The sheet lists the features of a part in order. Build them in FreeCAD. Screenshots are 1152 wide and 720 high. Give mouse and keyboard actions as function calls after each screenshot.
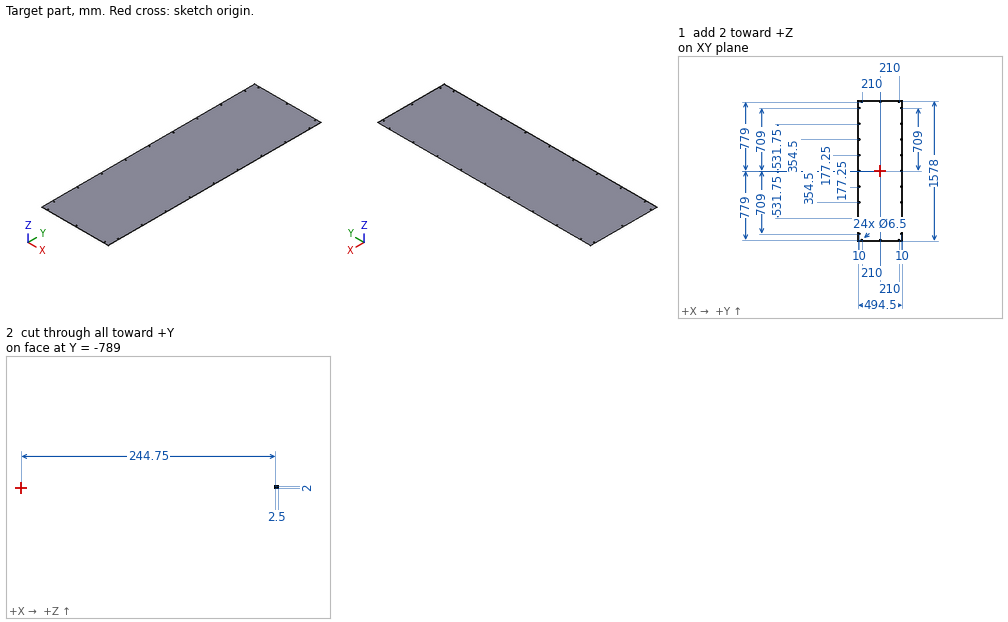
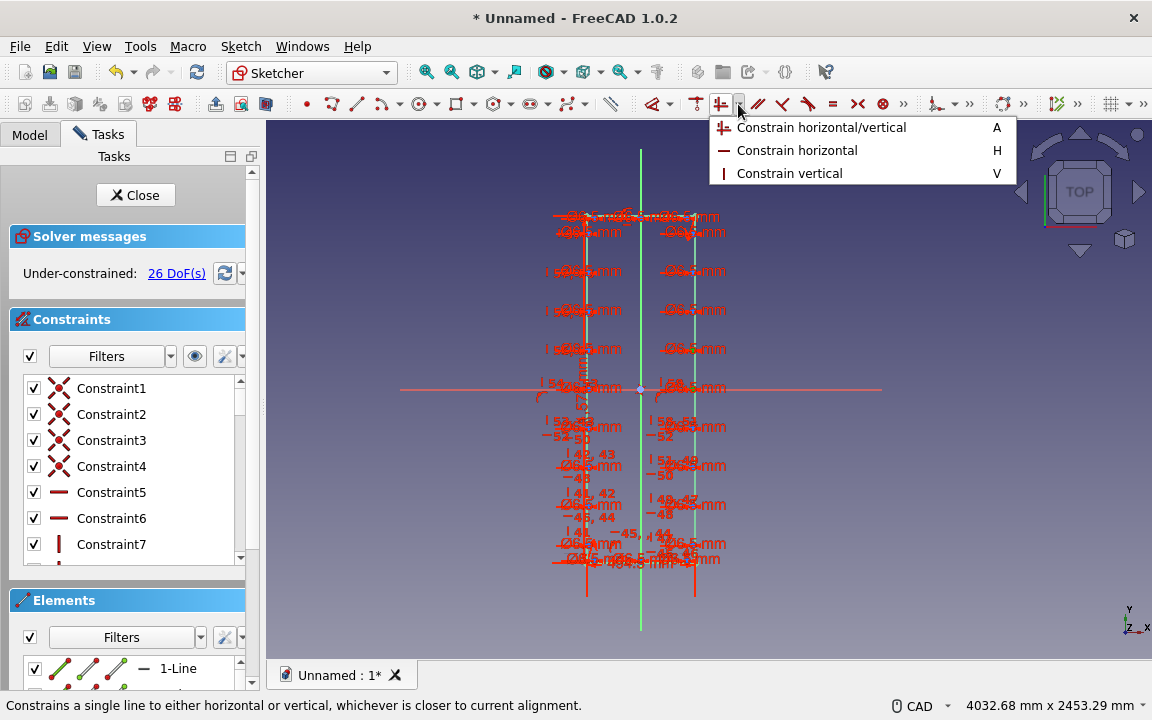
click(863, 174)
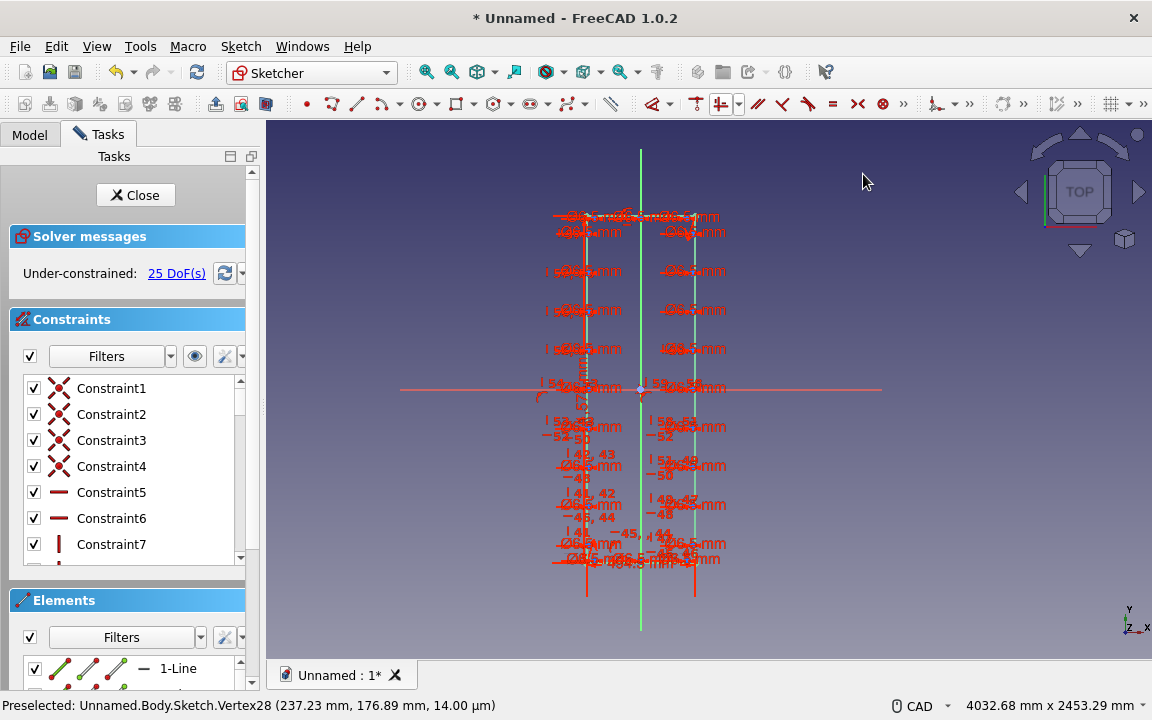
click(589, 351)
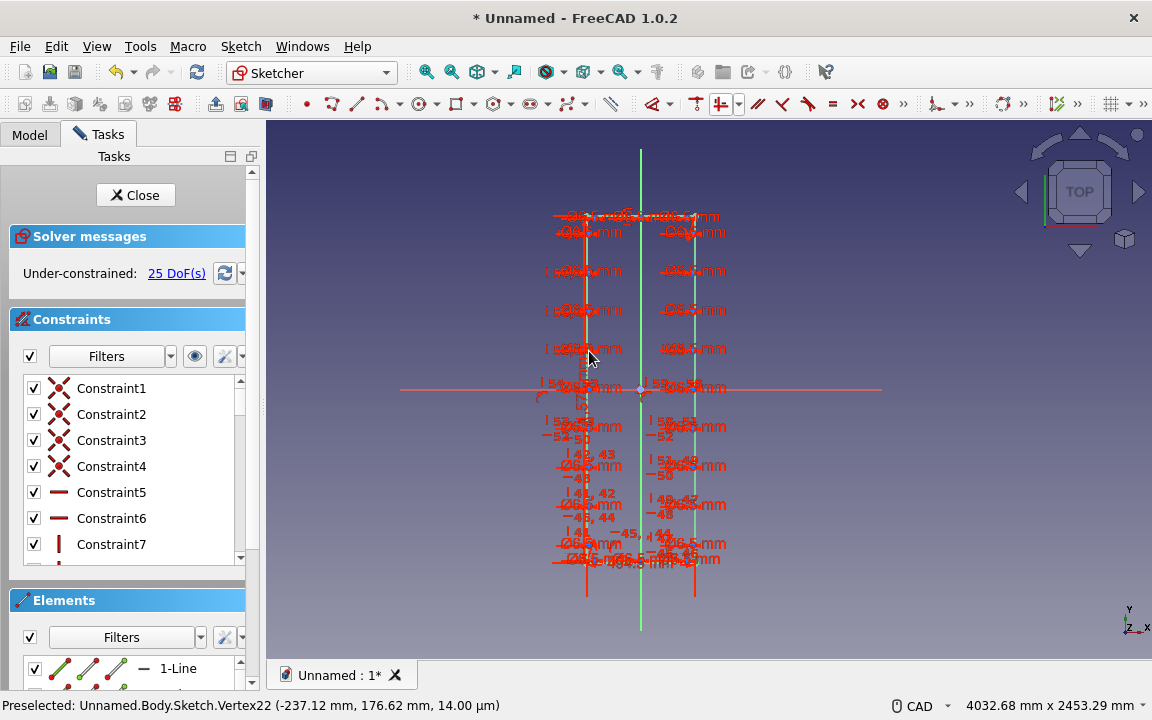
click(693, 351)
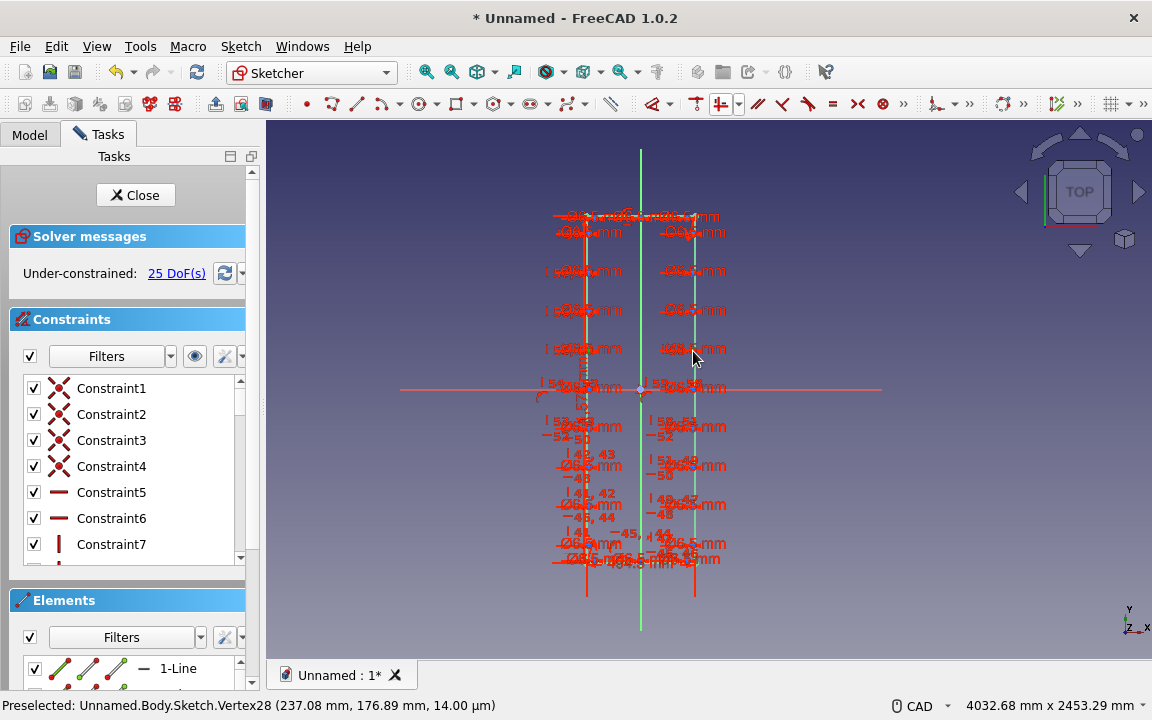
key(h)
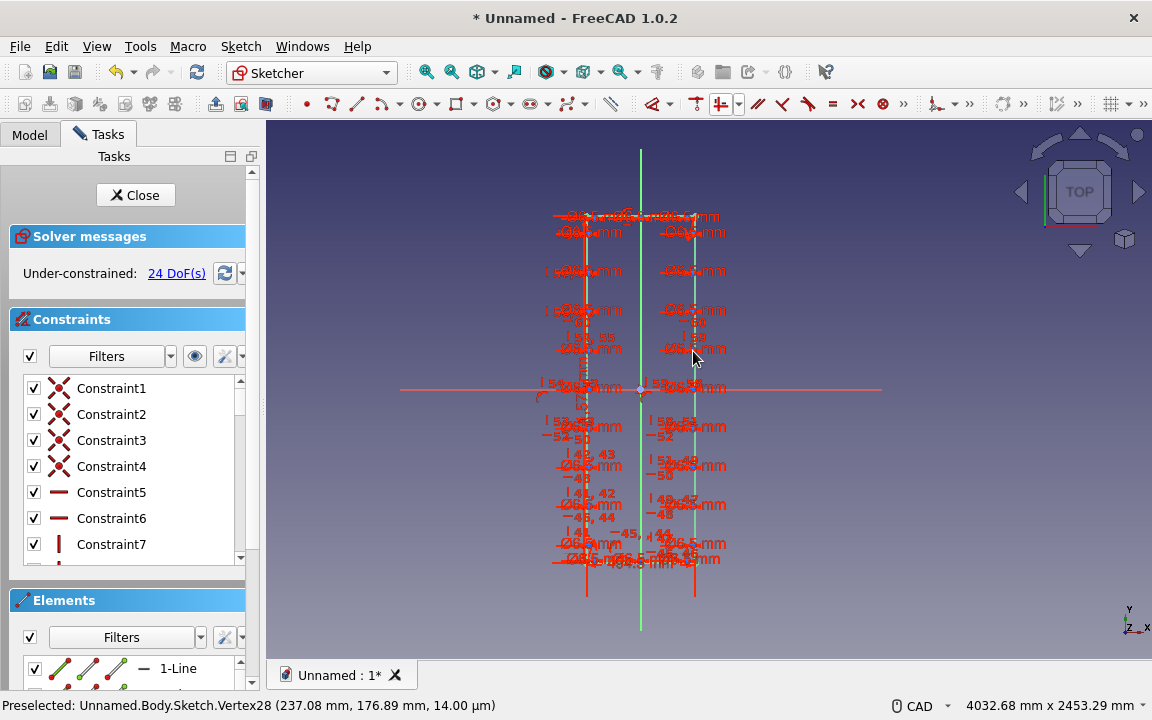
click(693, 351)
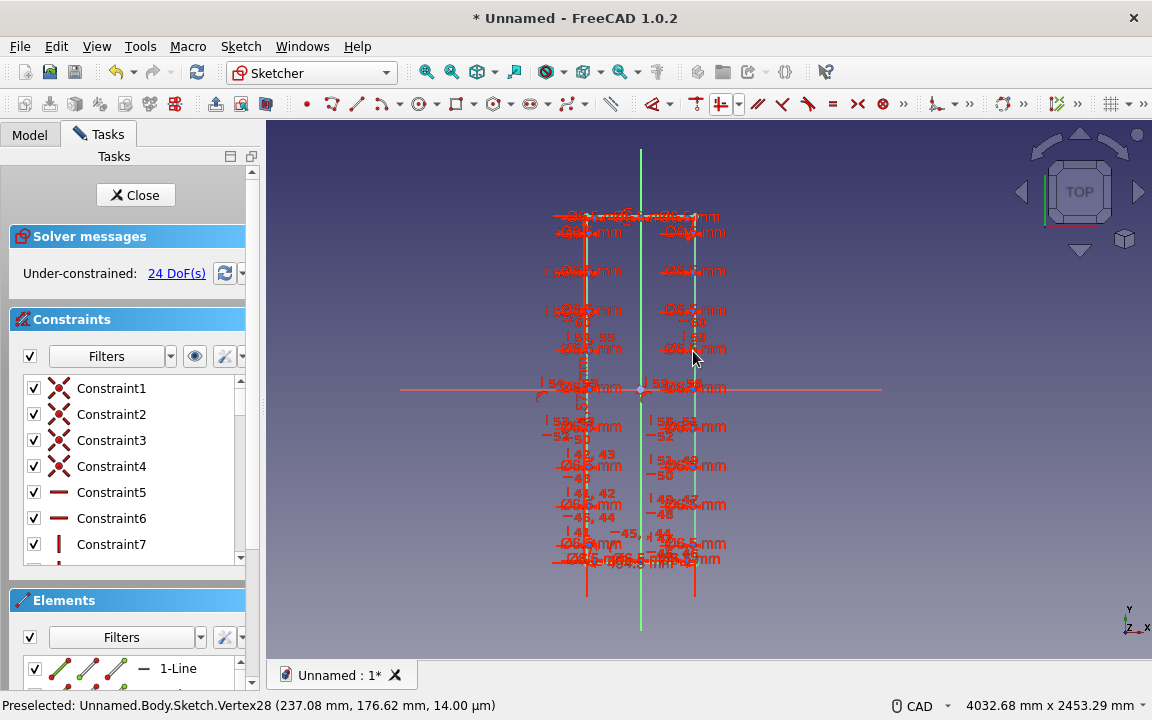
click(693, 312)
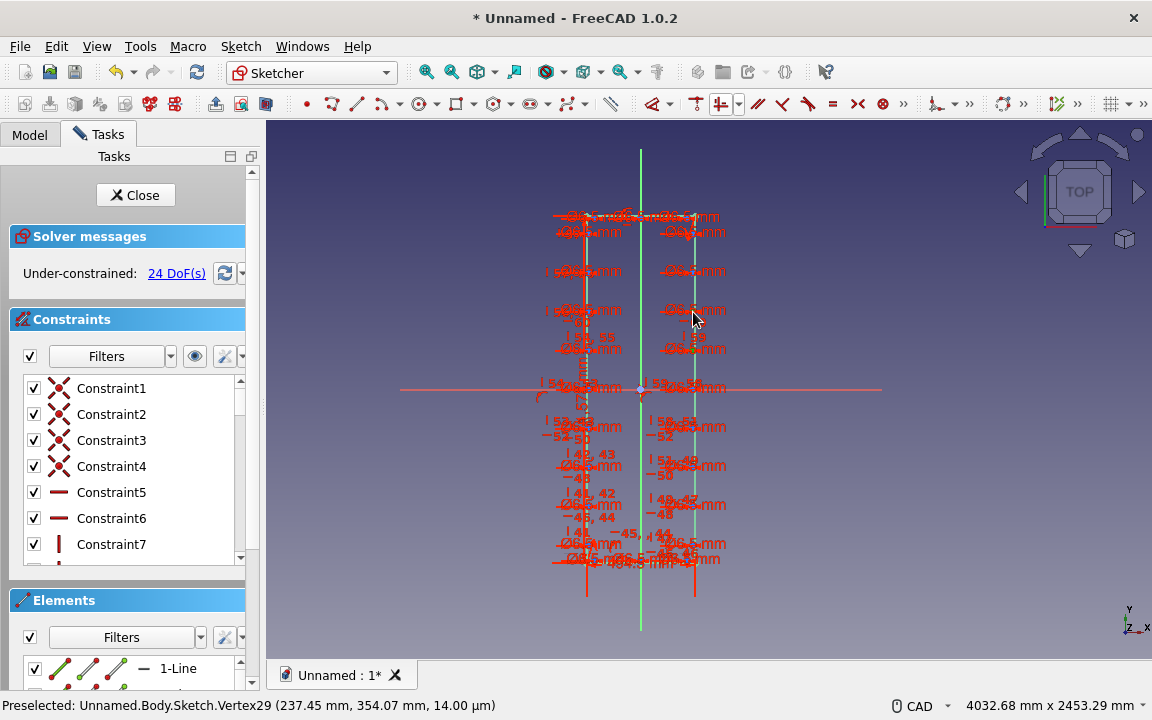
click(738, 104)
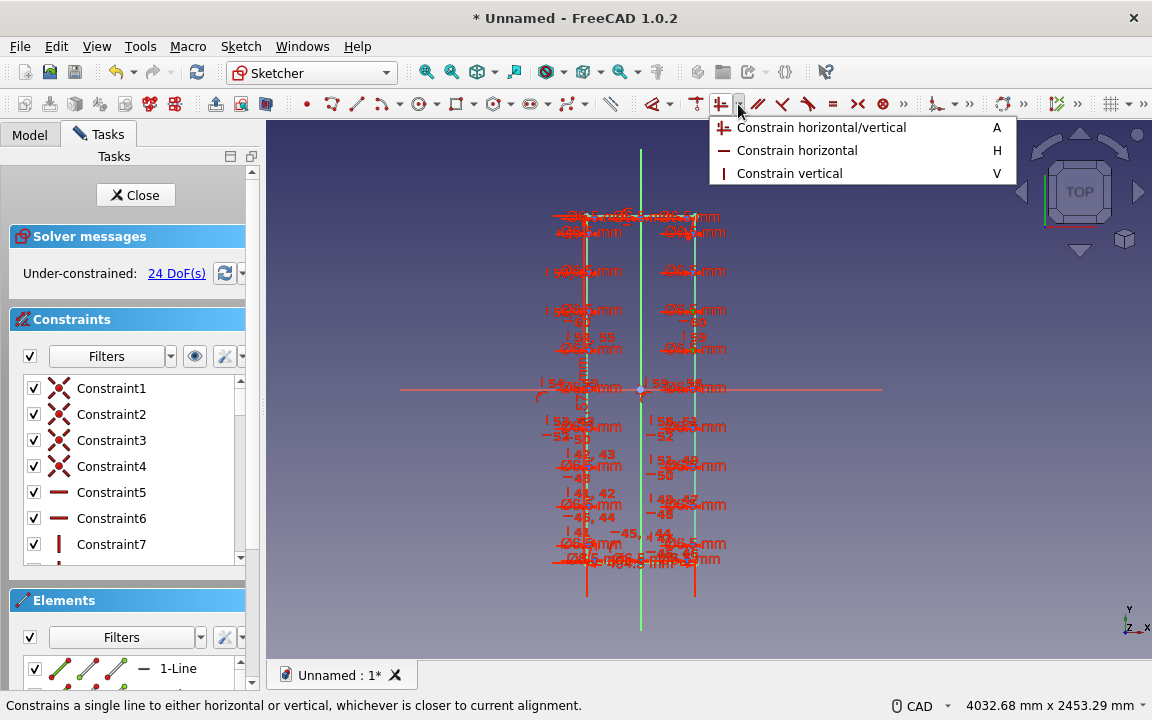
click(863, 174)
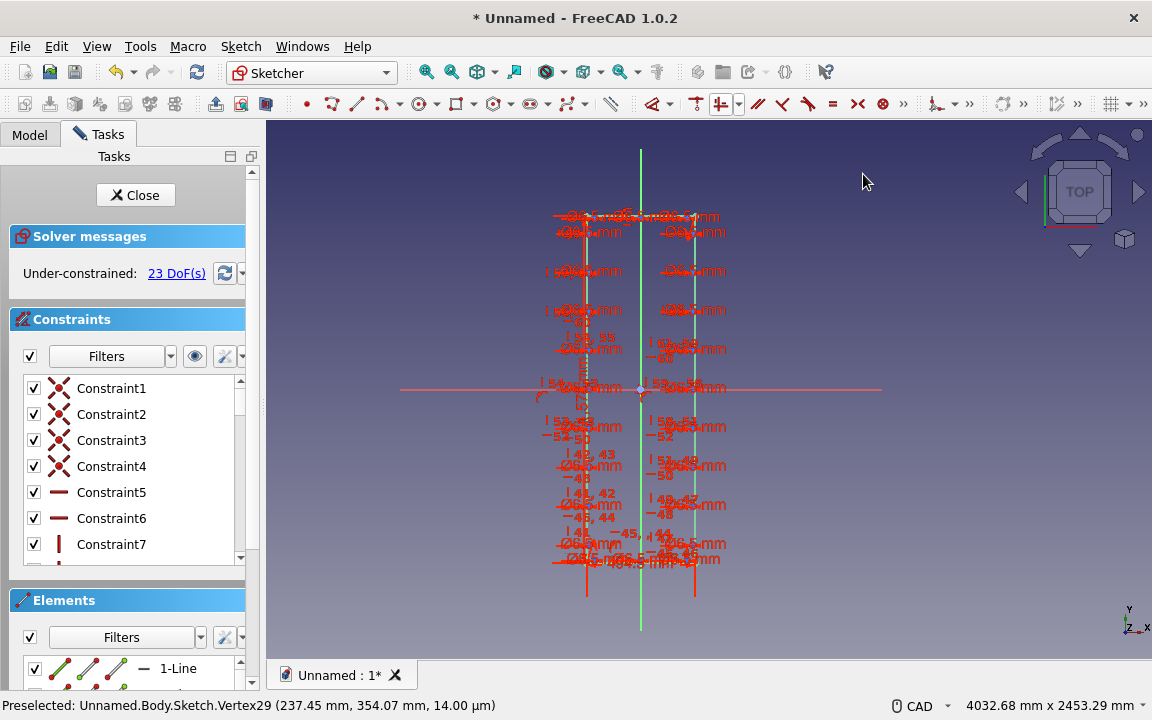
click(589, 312)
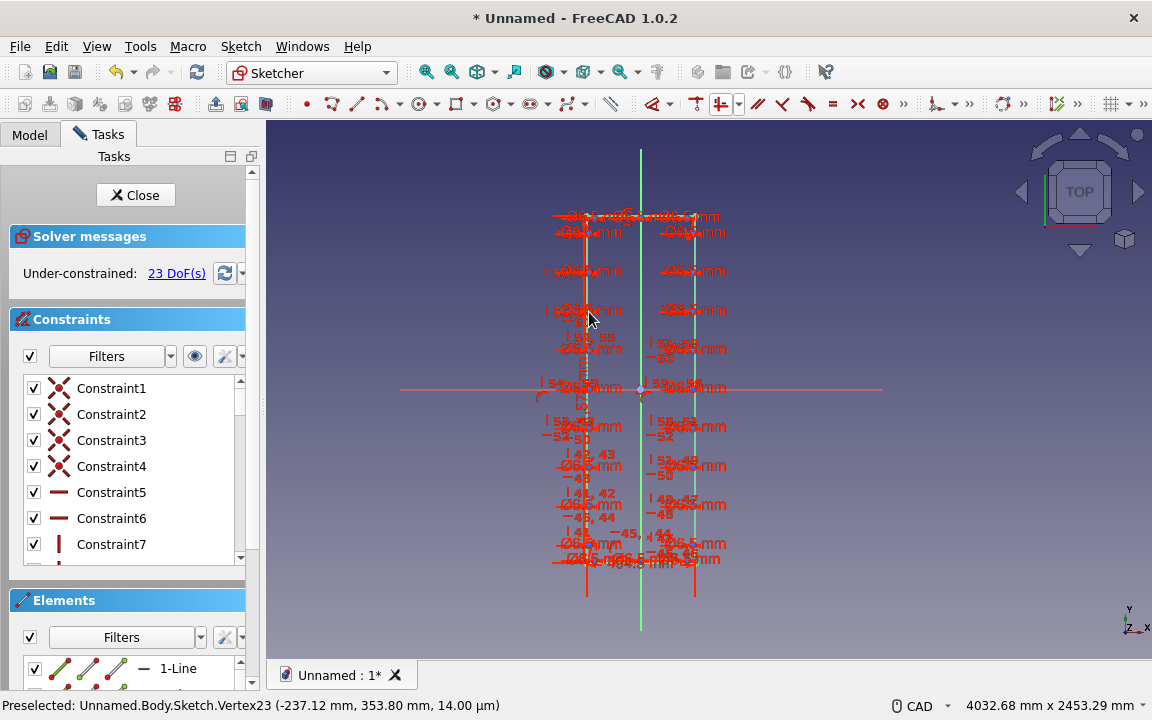
click(693, 312)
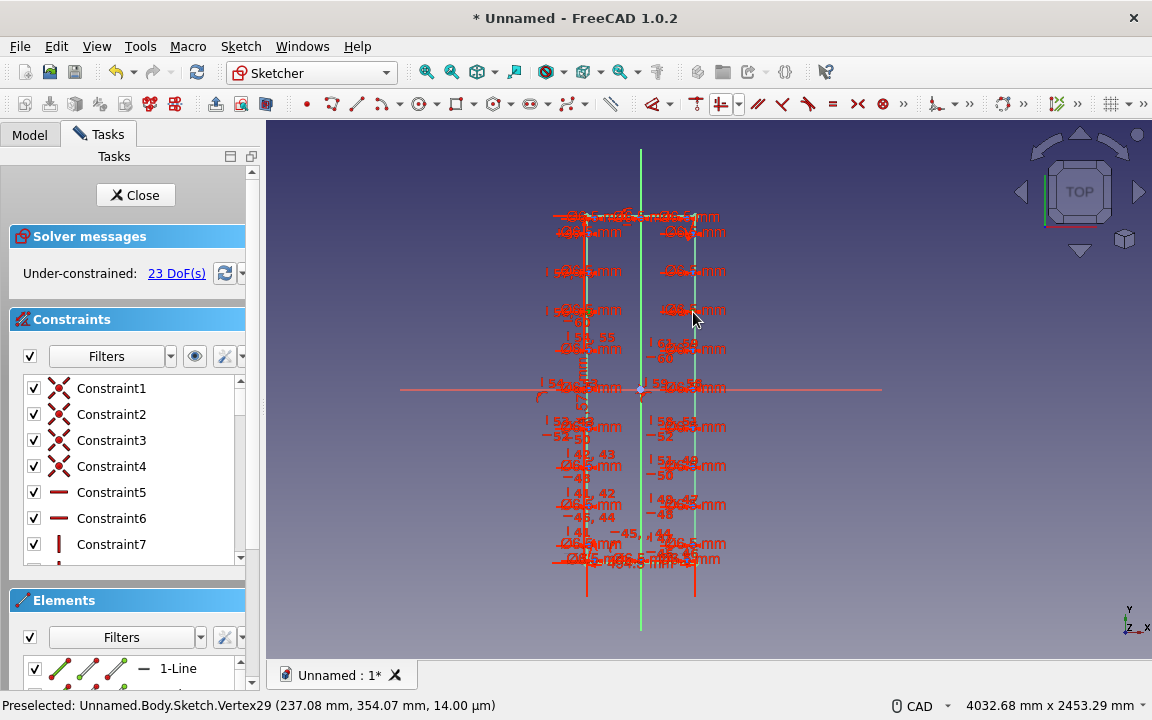
click(738, 104)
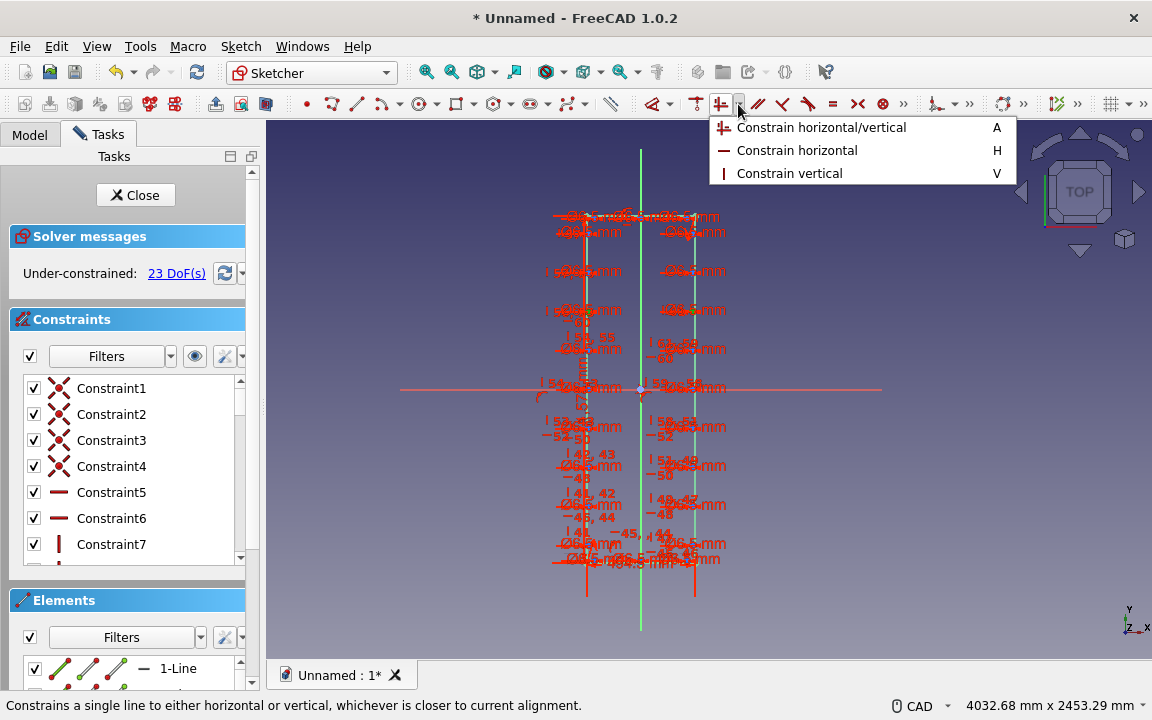
click(863, 150)